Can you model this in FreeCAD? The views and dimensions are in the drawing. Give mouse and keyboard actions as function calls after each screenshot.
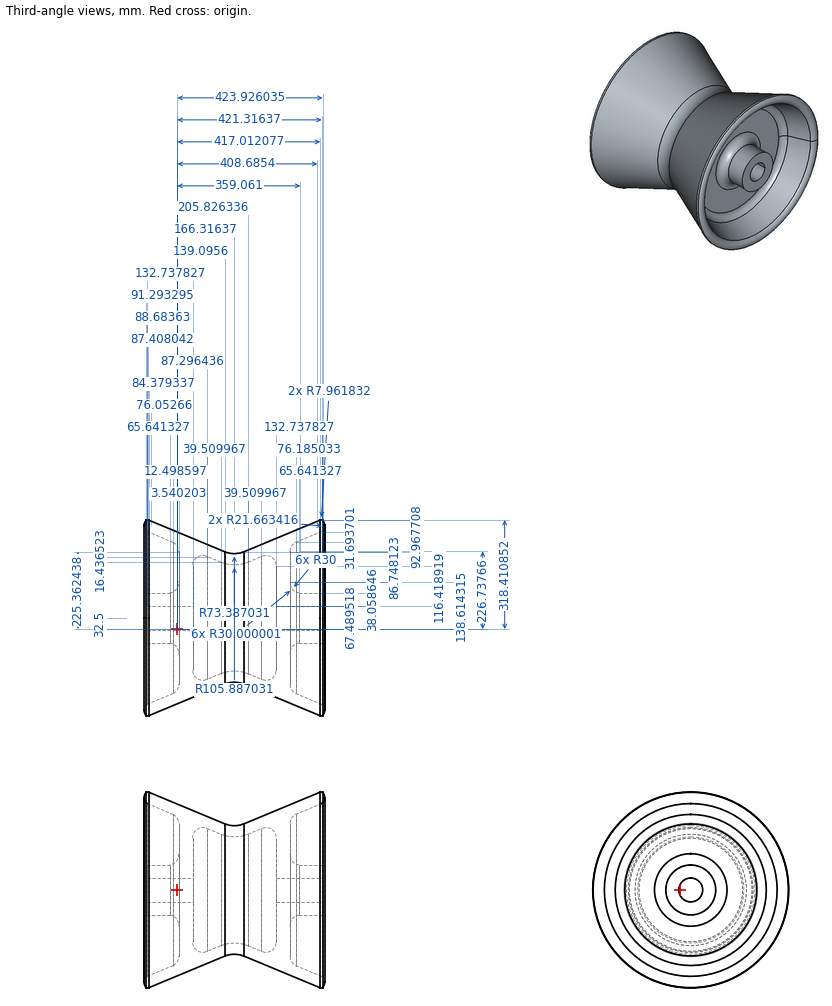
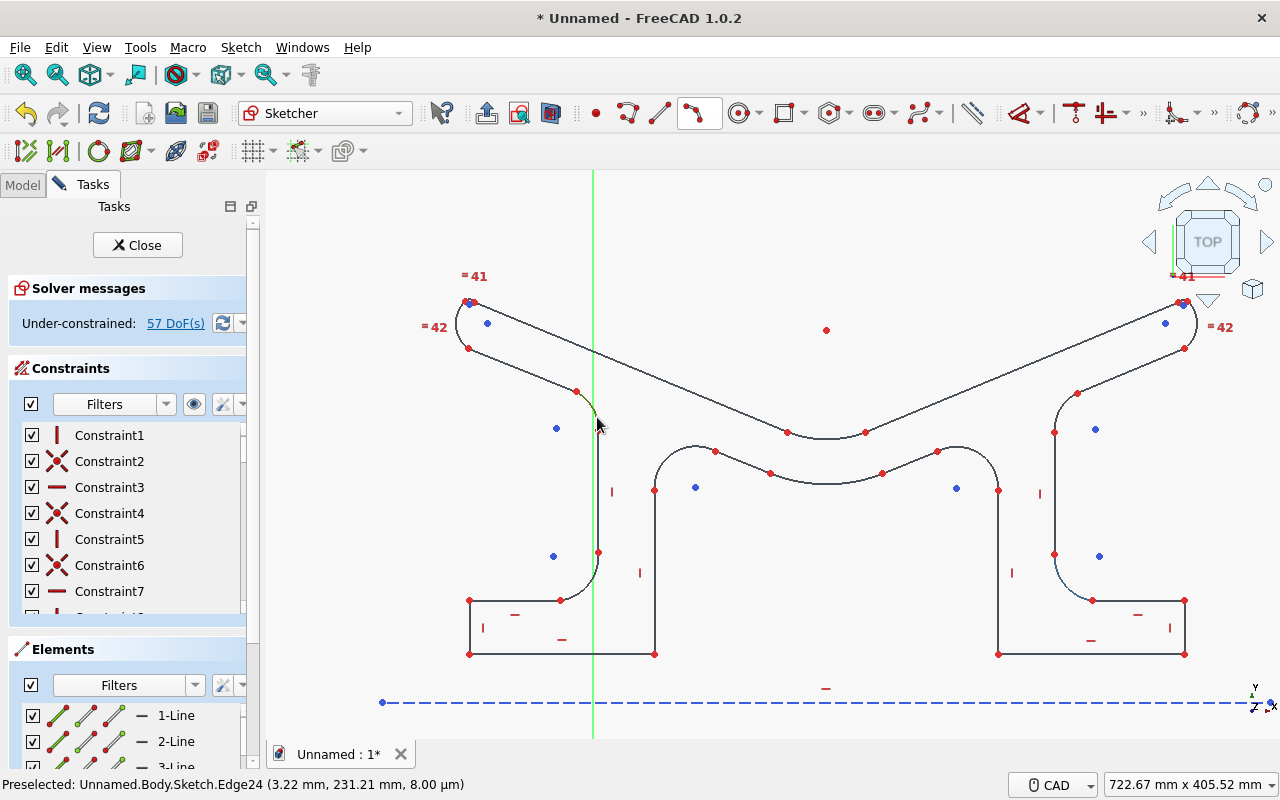
click(579, 593)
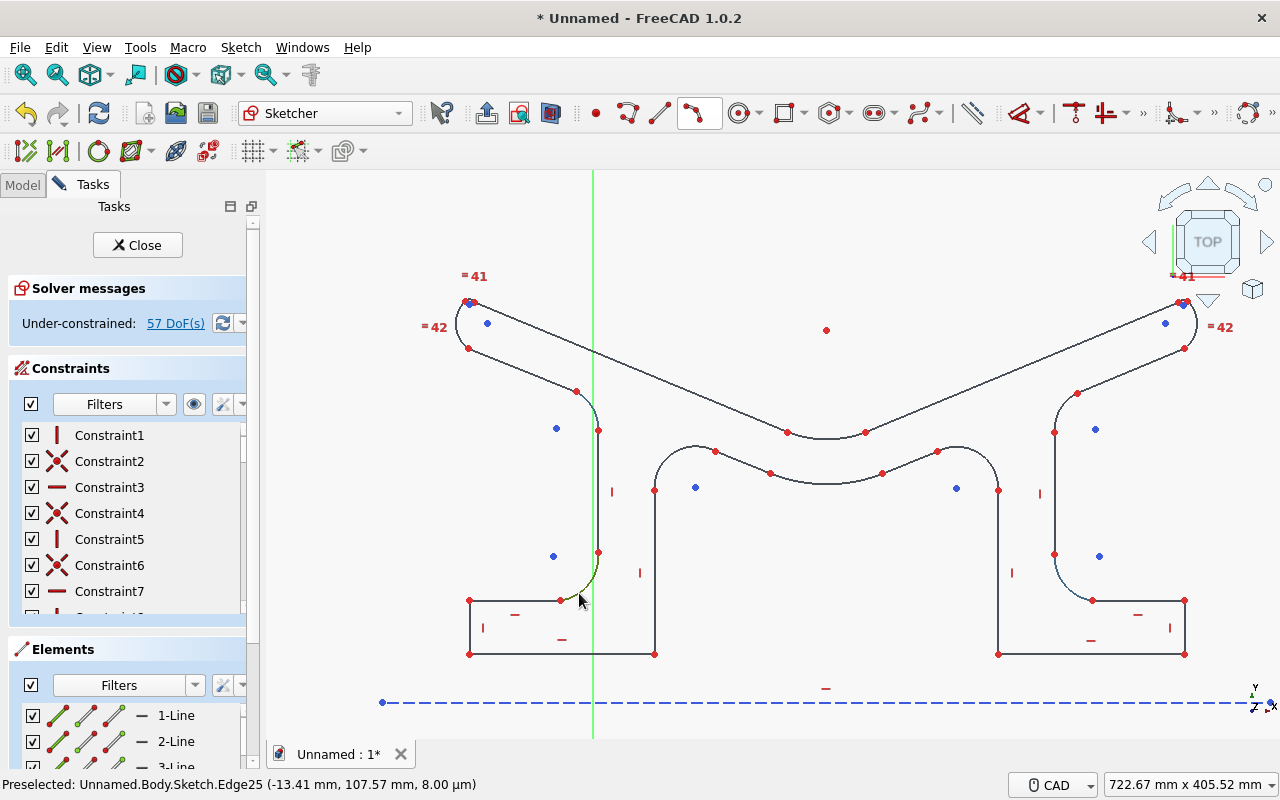
click(690, 447)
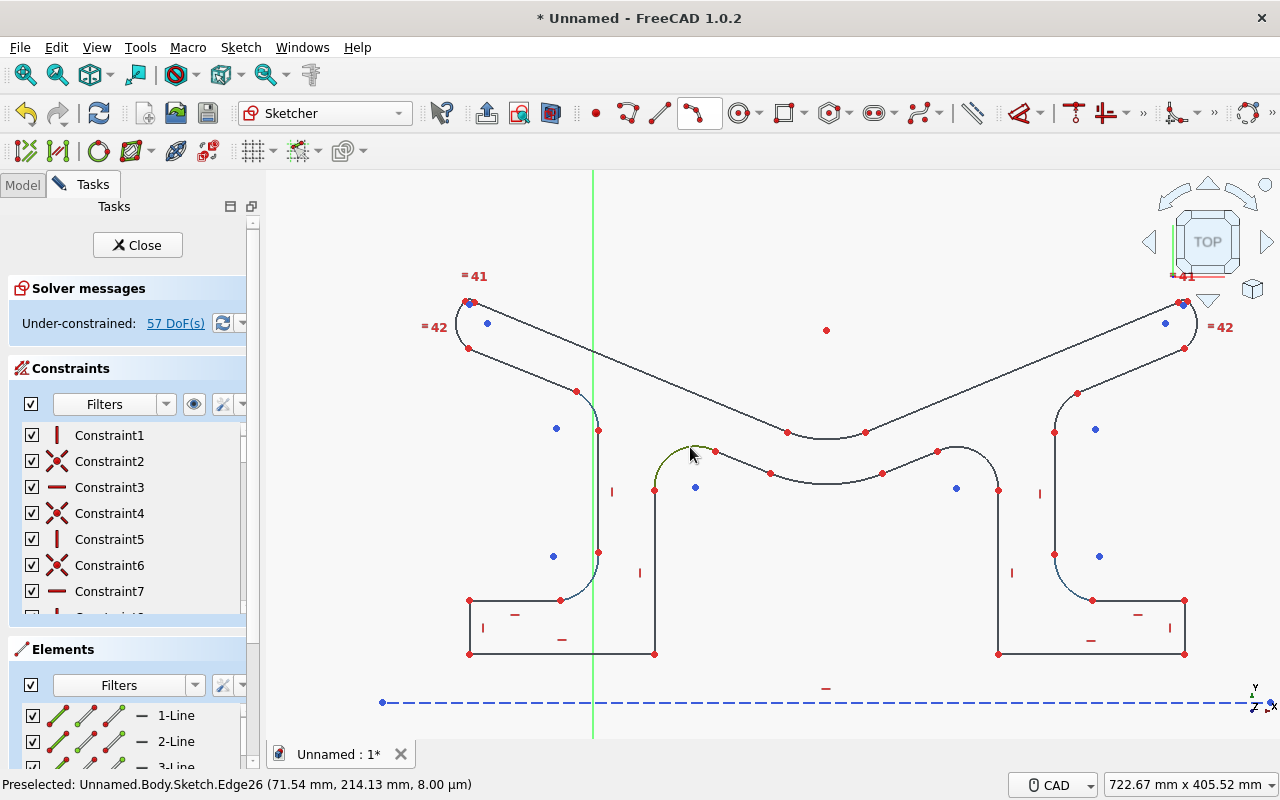
click(991, 466)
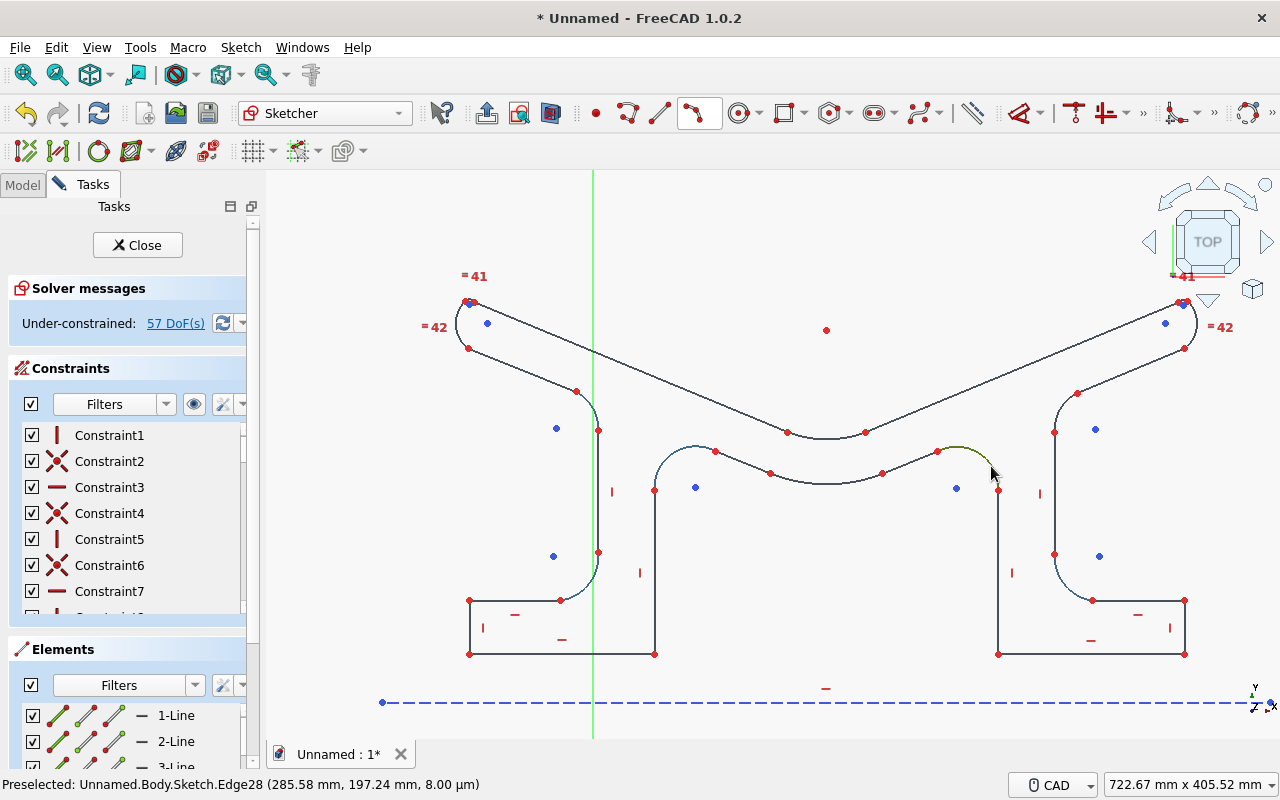
key(e)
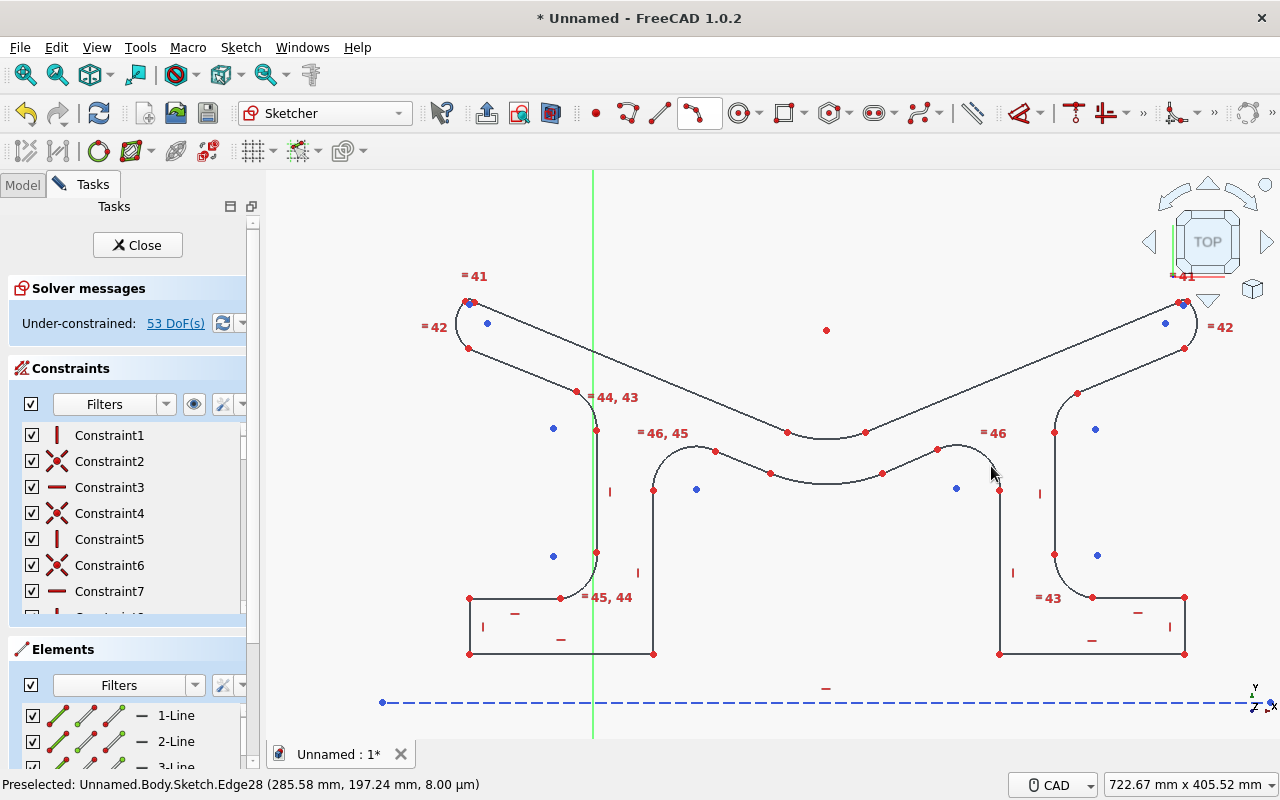
click(1020, 114)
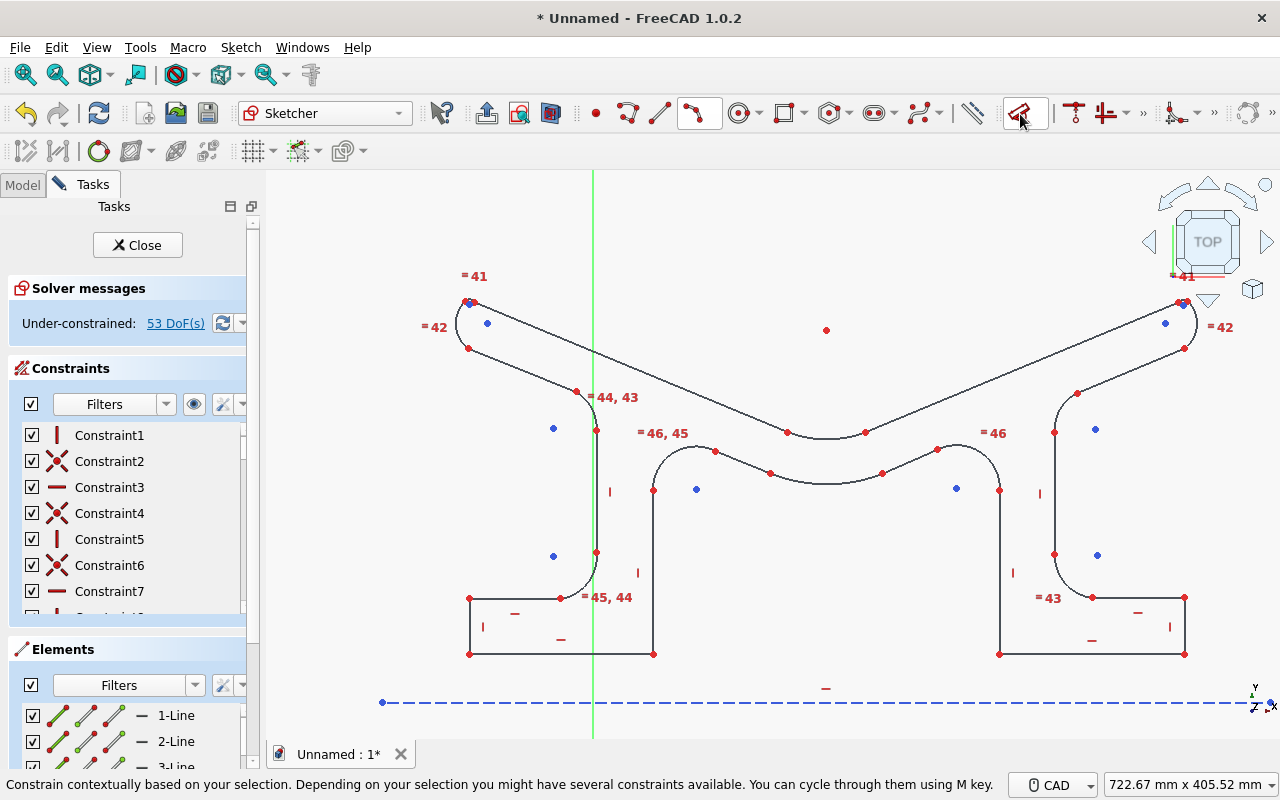
click(1058, 573)
click(1029, 586)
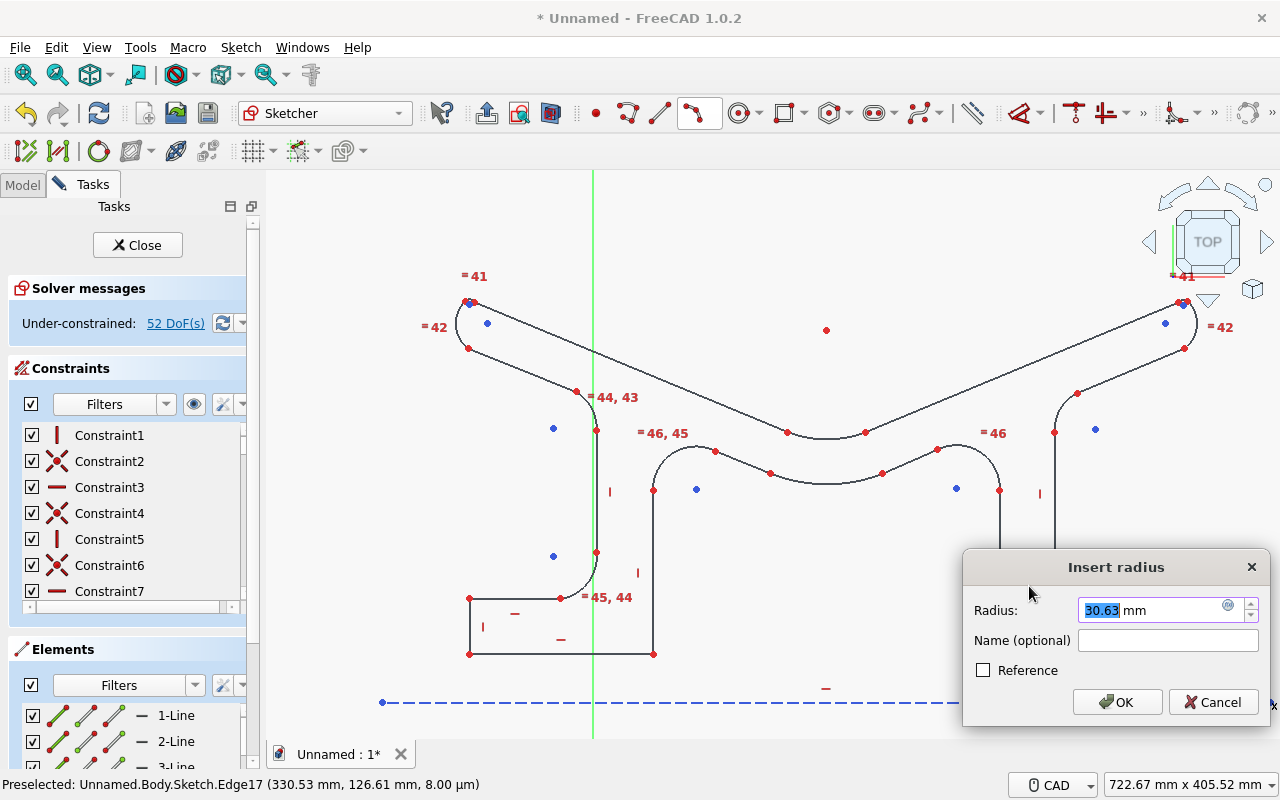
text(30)
key(Return)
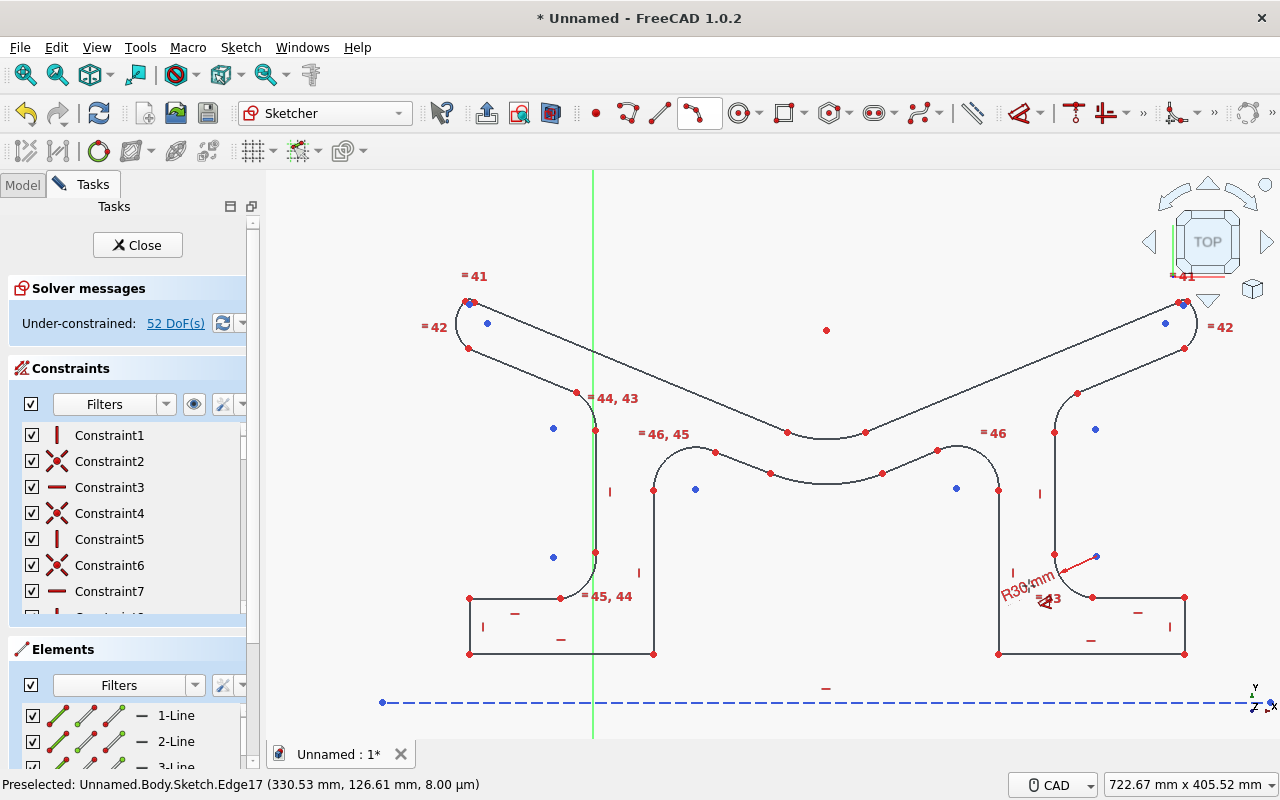
click(1066, 402)
click(1043, 380)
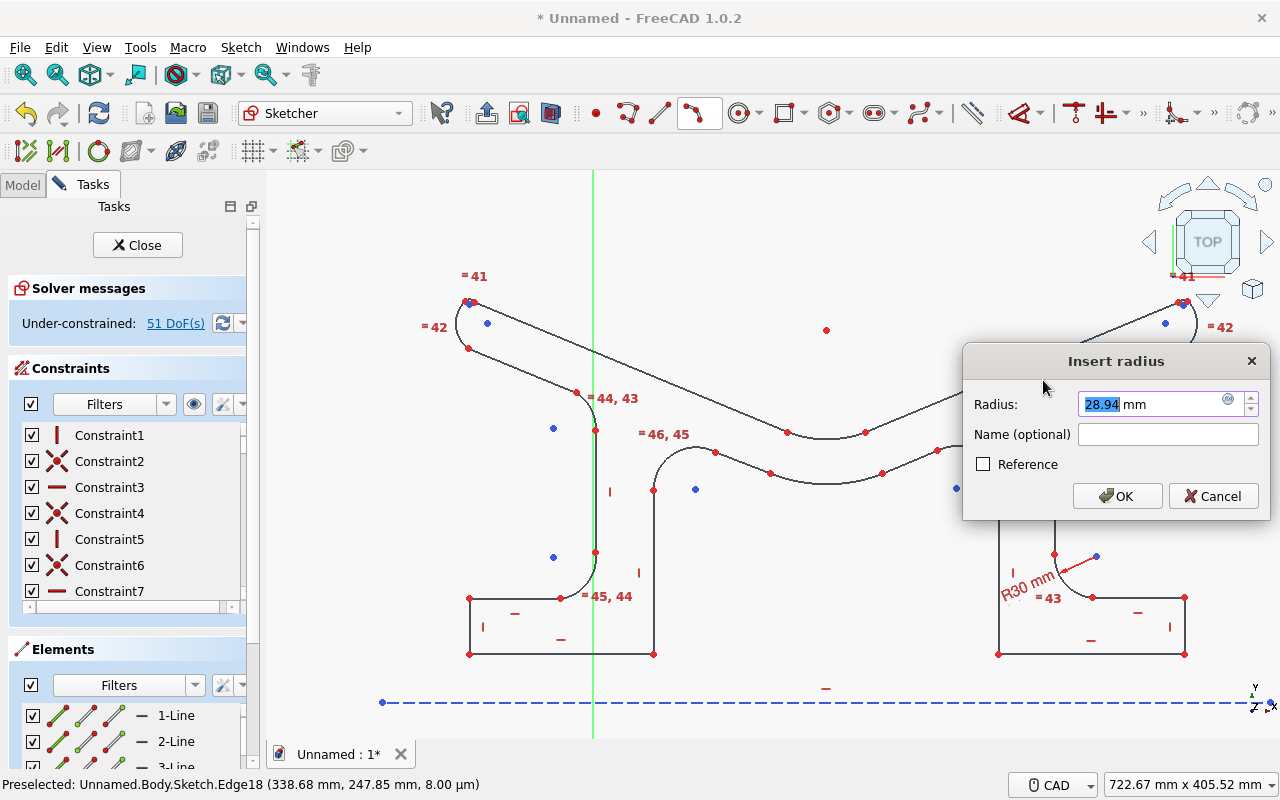
text(30.000001)
key(Return)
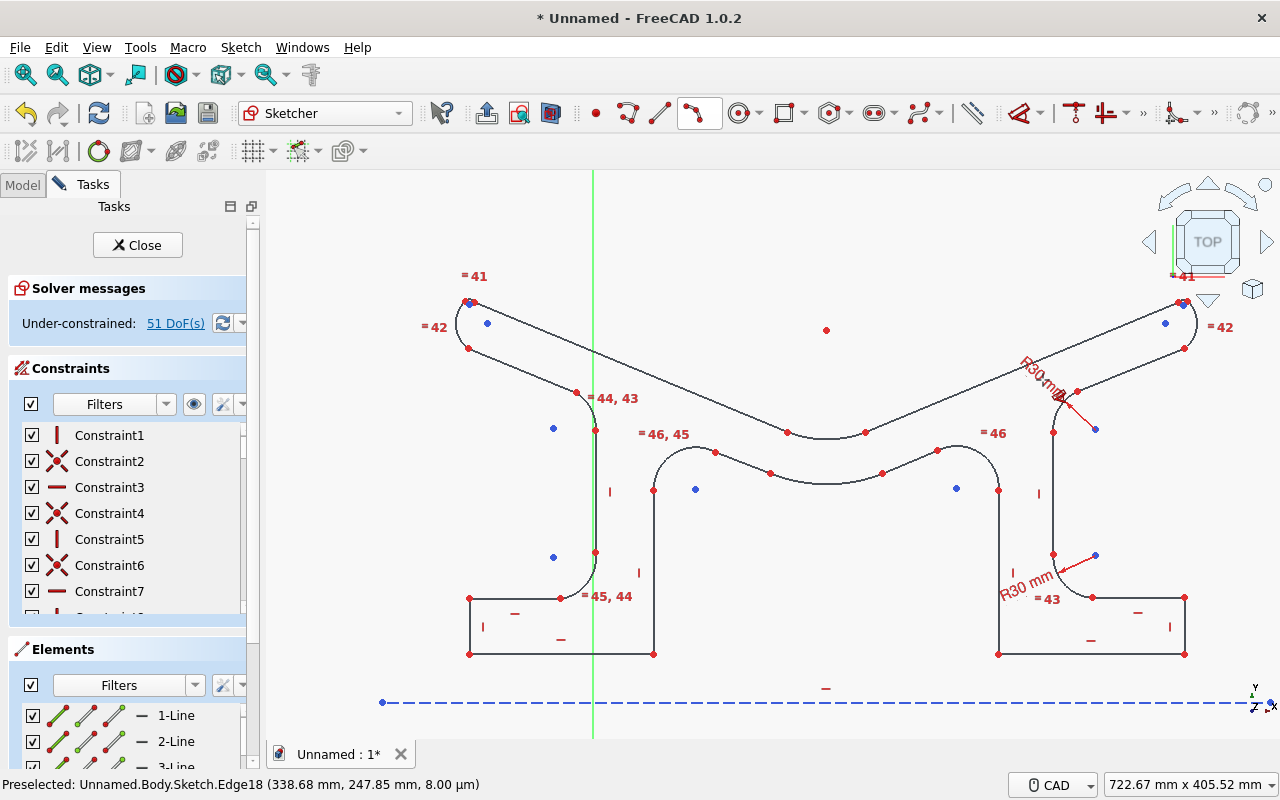
scroll(456, 315, down, 2)